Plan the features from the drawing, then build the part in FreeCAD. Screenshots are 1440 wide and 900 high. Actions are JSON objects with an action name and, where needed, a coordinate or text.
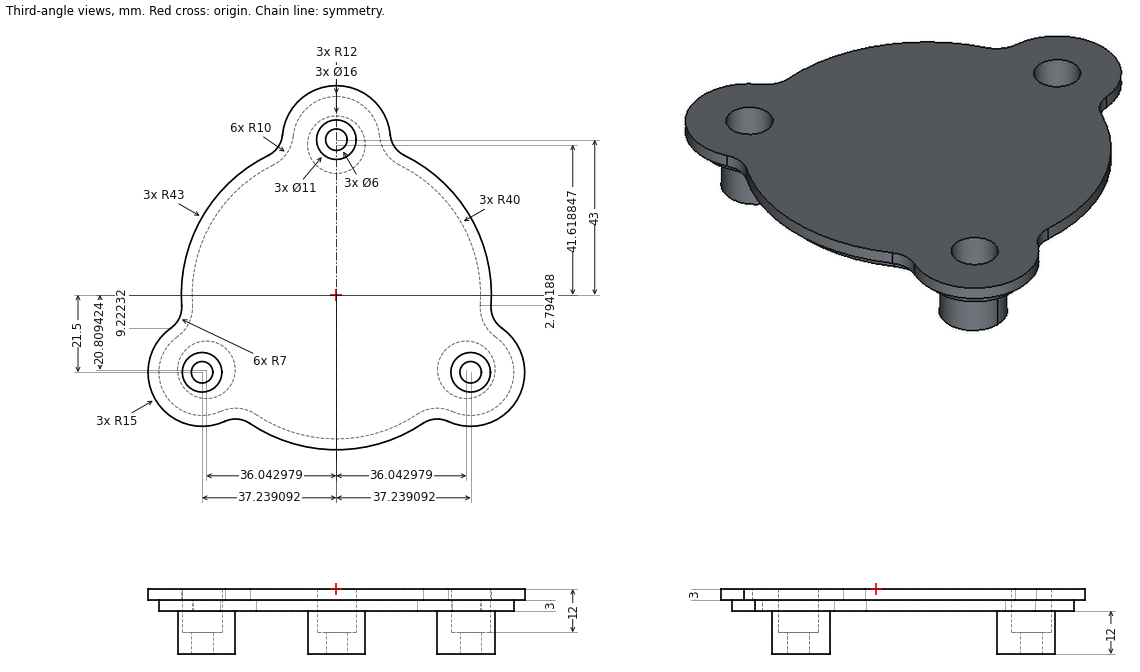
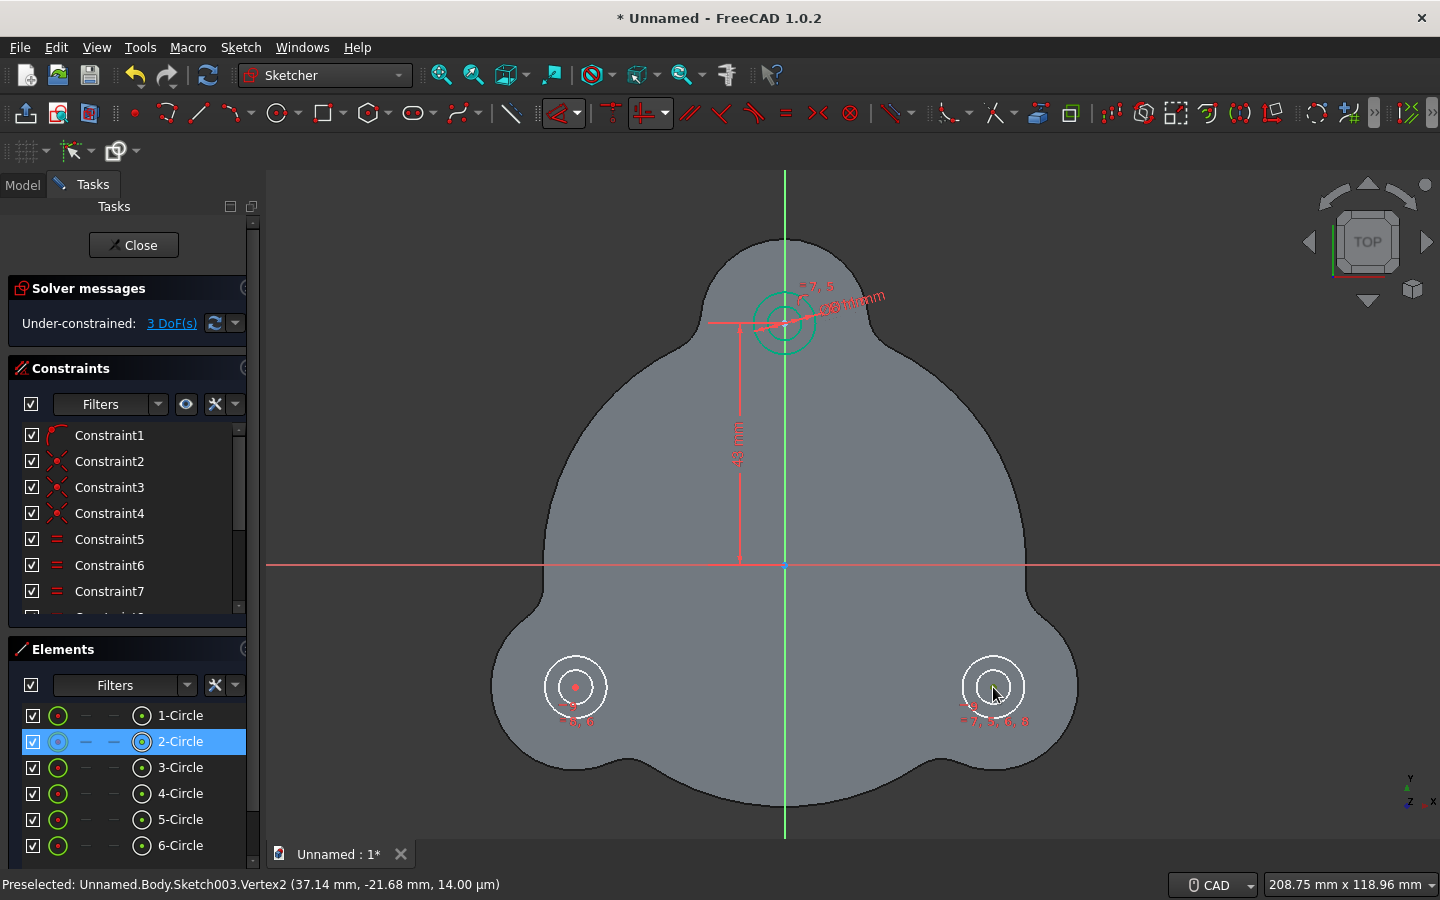
{"action": "left_click", "coordinate": [580, 114]}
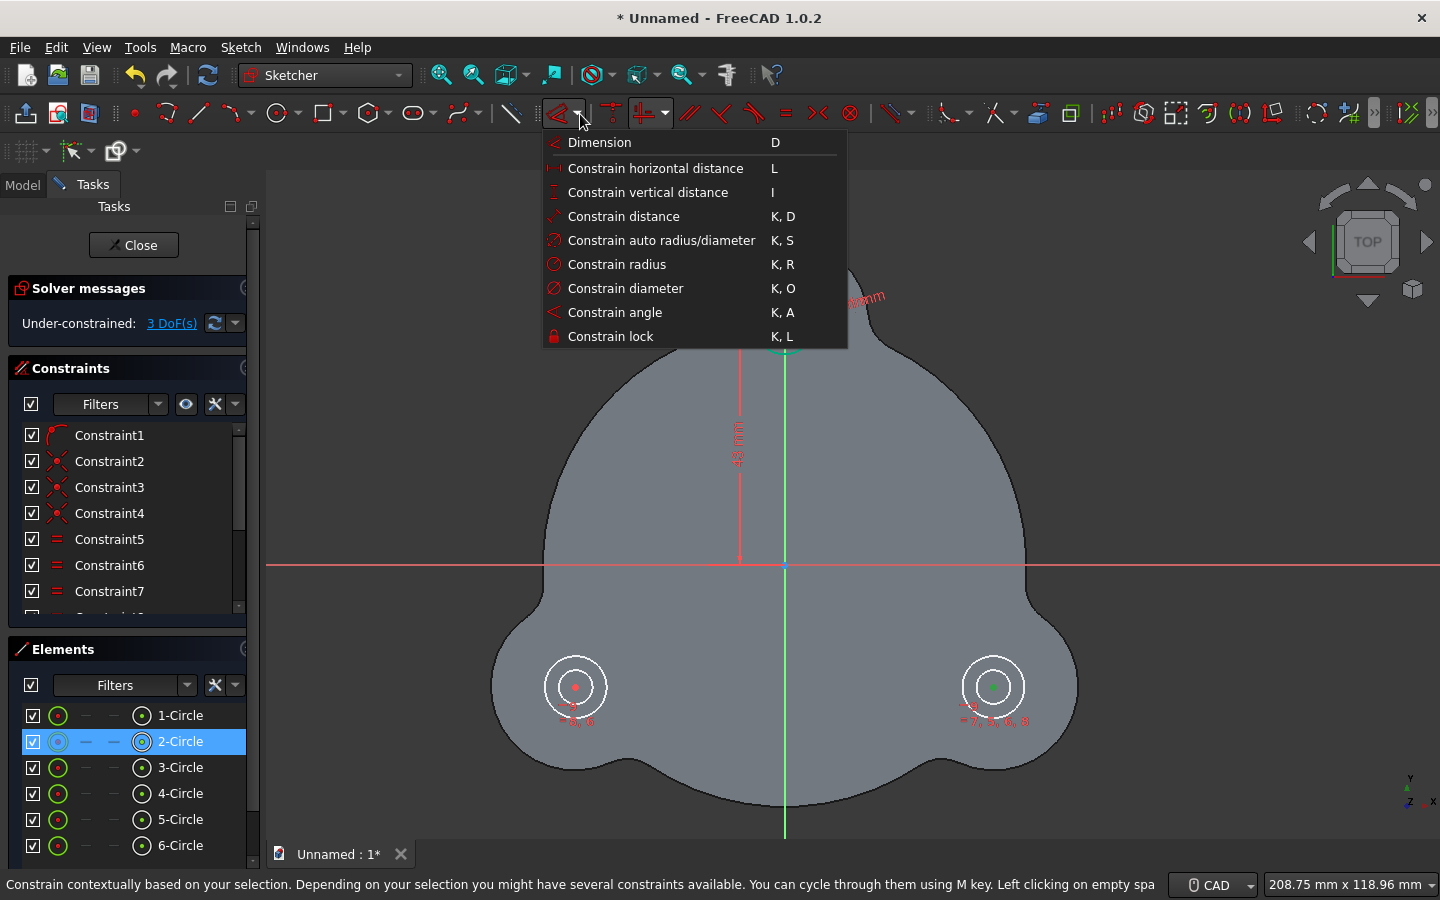
{"action": "left_click", "coordinate": [695, 192]}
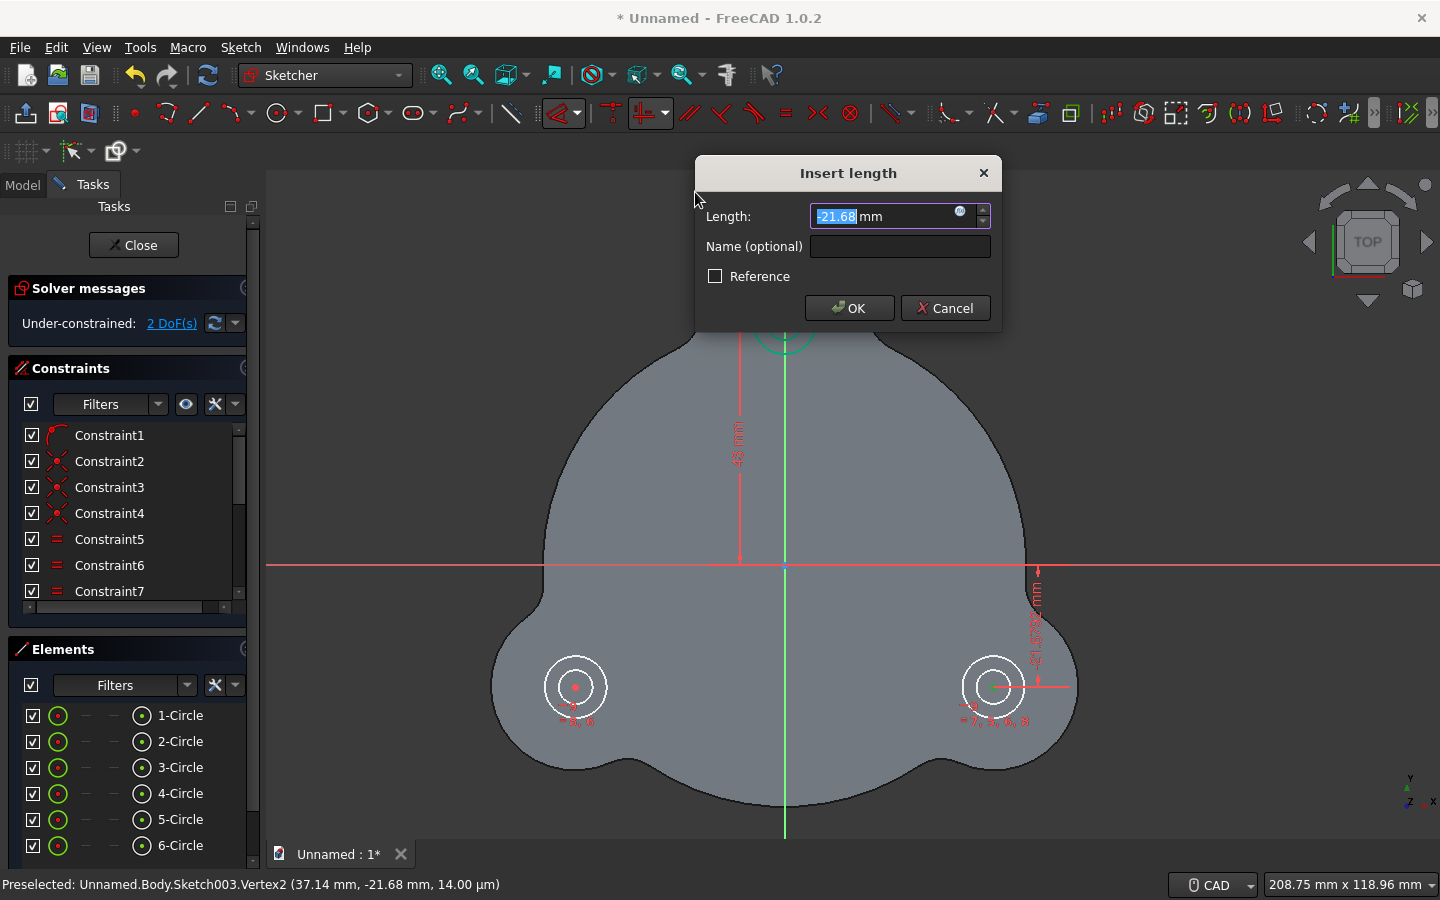
{"action": "type", "text": "-21.5"}
{"action": "key", "text": "Return"}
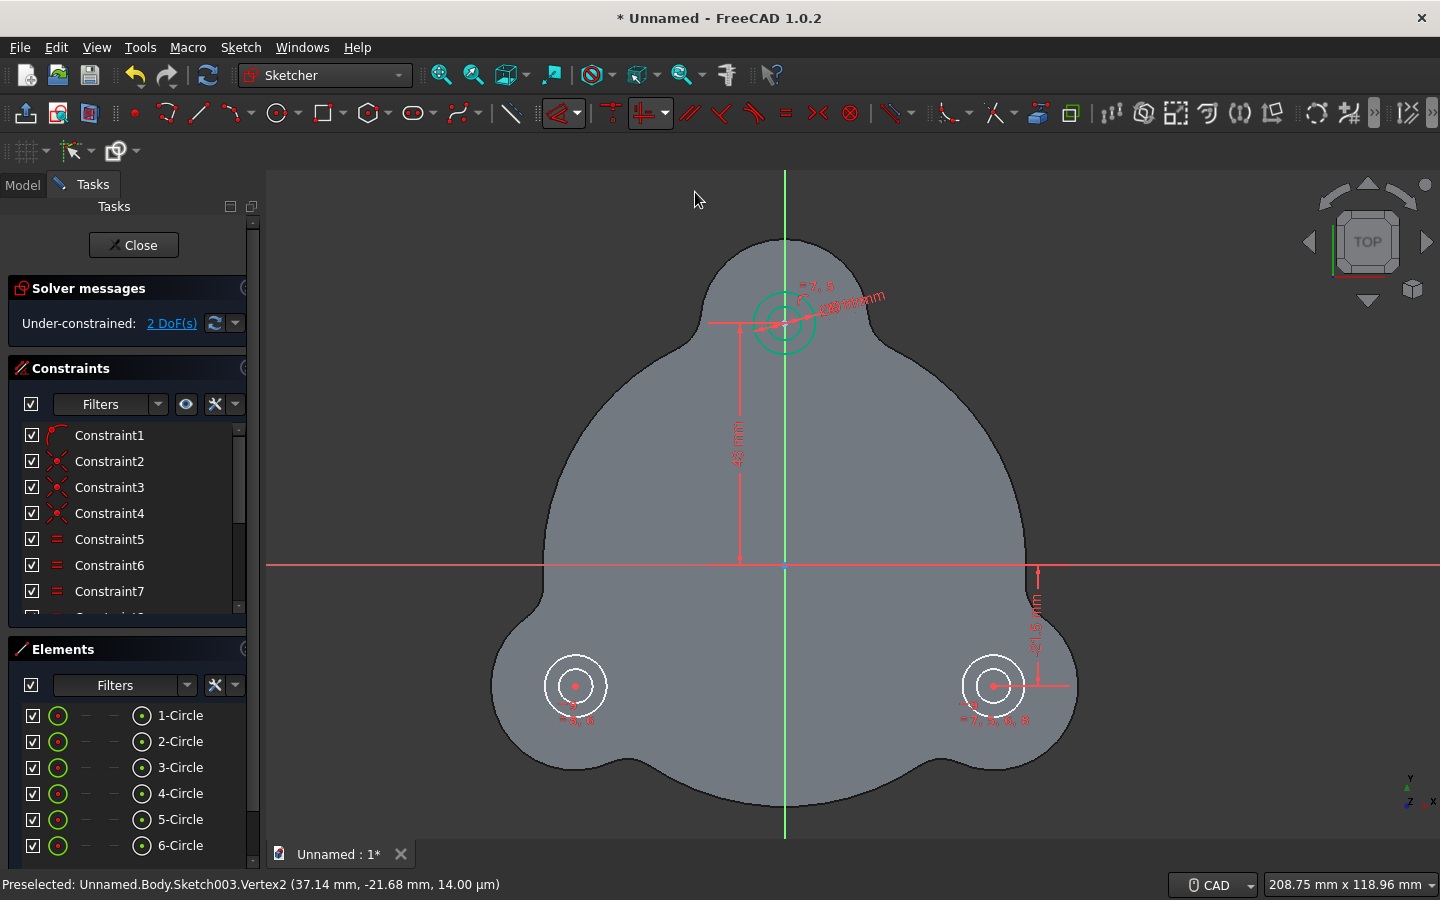
{"action": "left_click", "coordinate": [993, 686]}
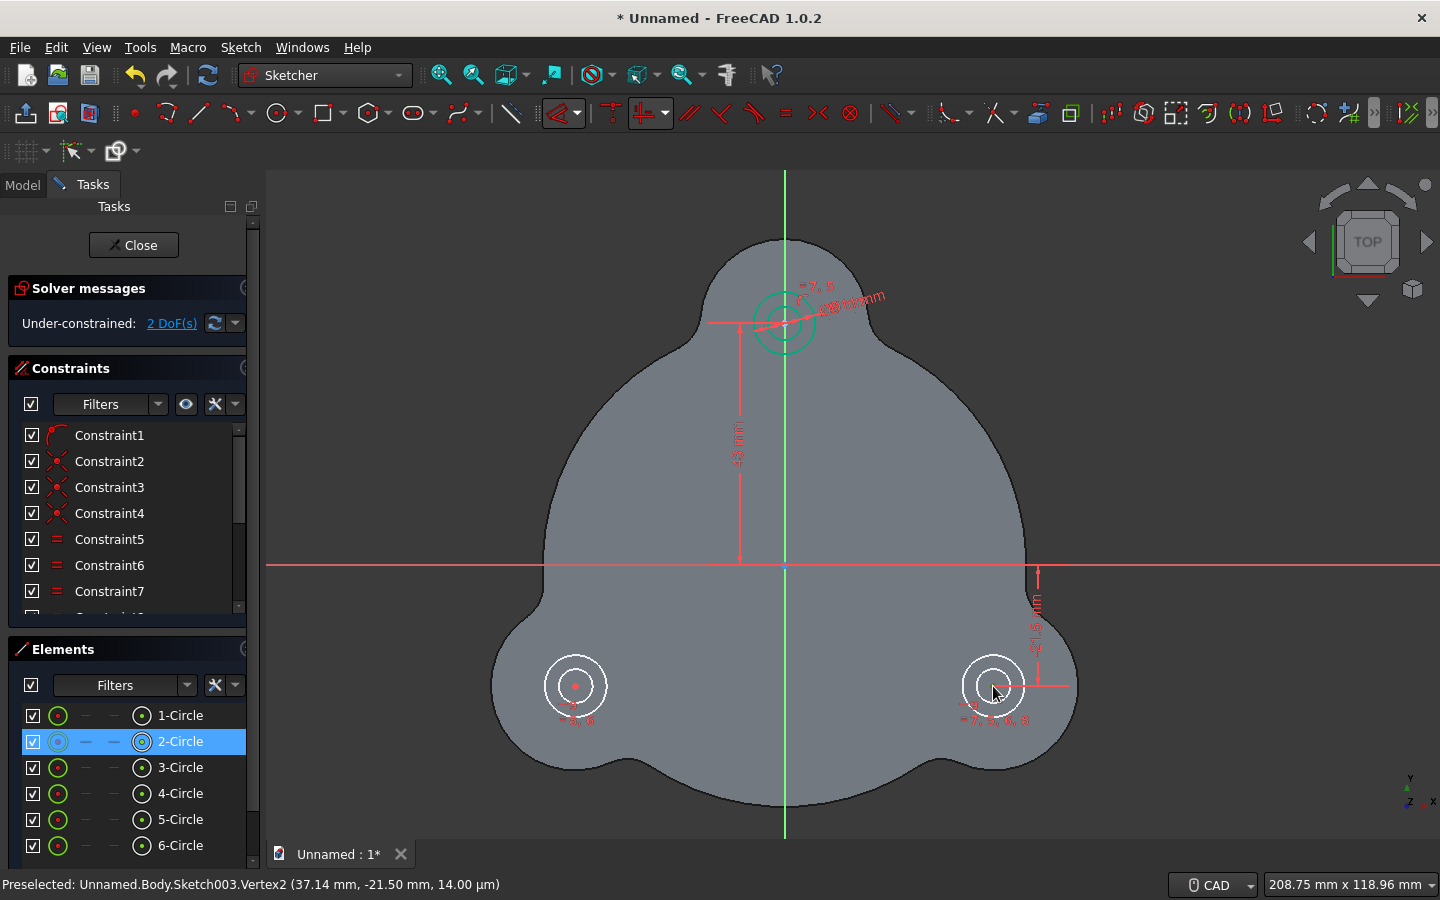
{"action": "left_click", "coordinate": [580, 114]}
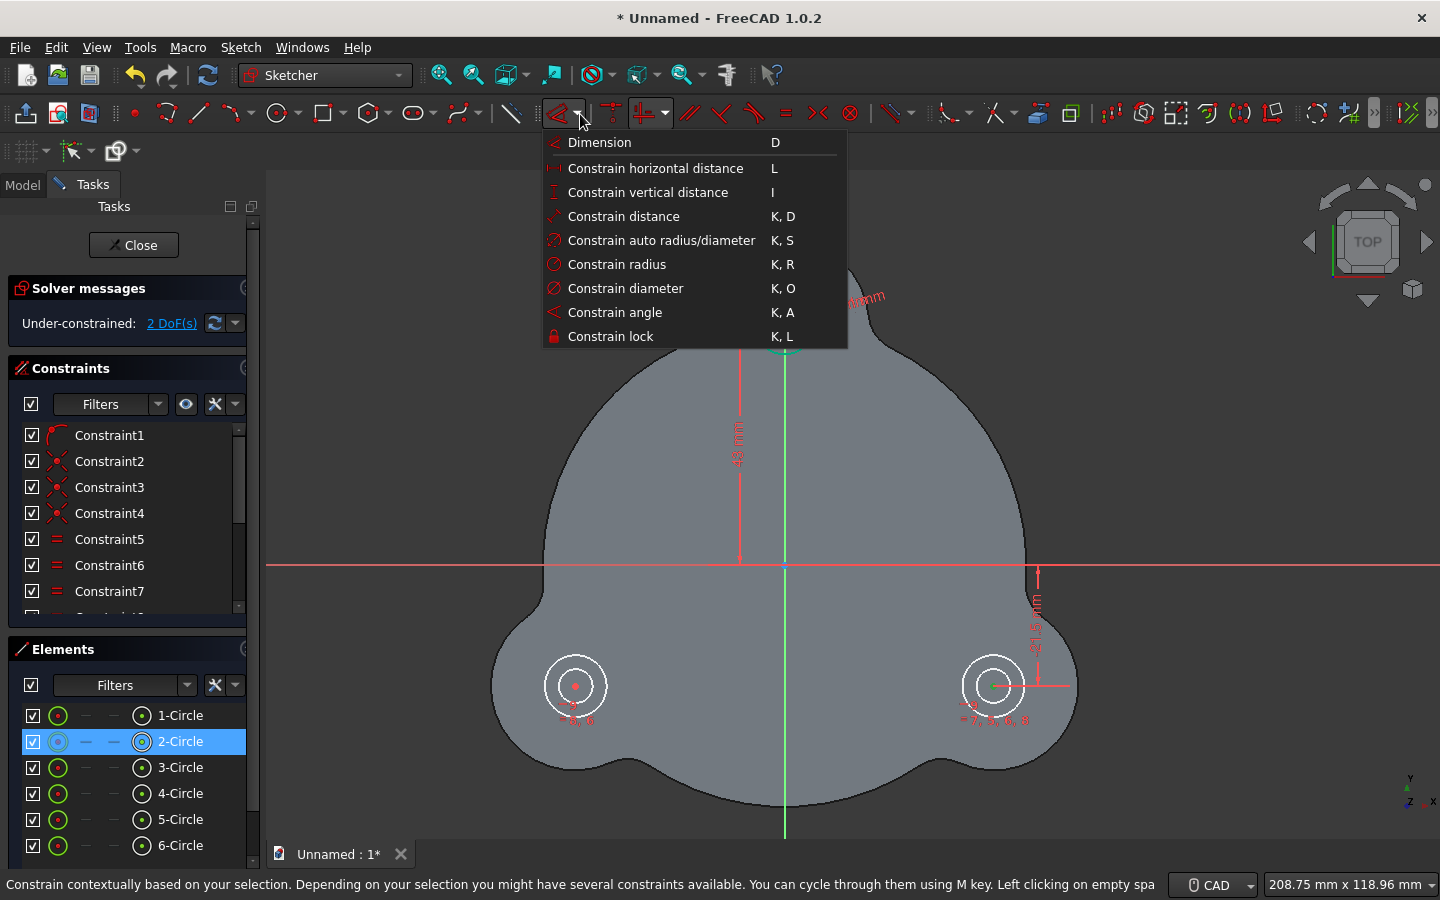
{"action": "left_click", "coordinate": [695, 168]}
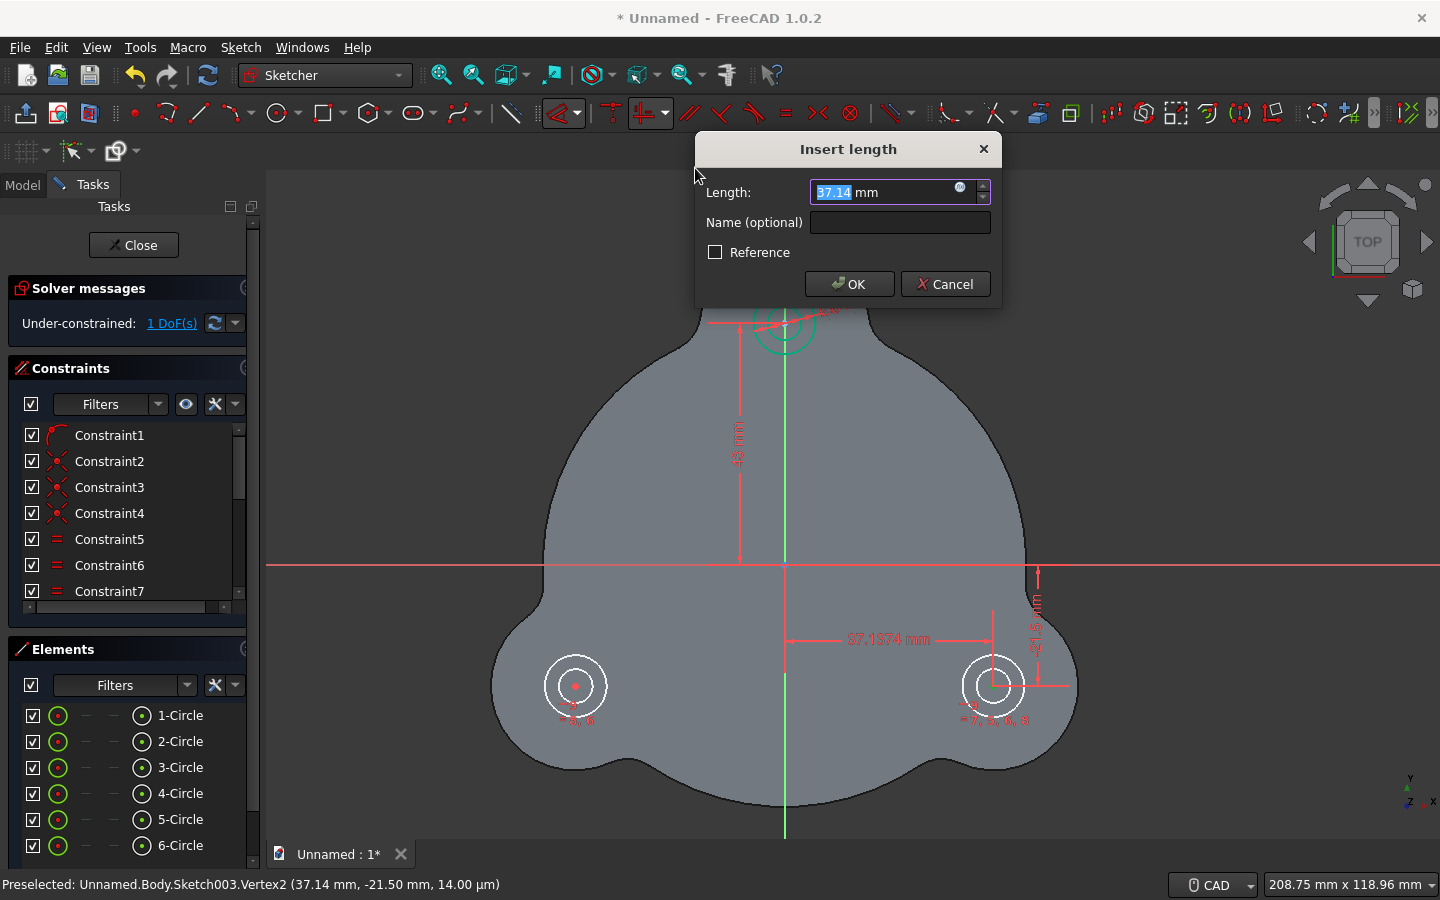
{"action": "type", "text": "37.239092"}
{"action": "key", "text": "Return"}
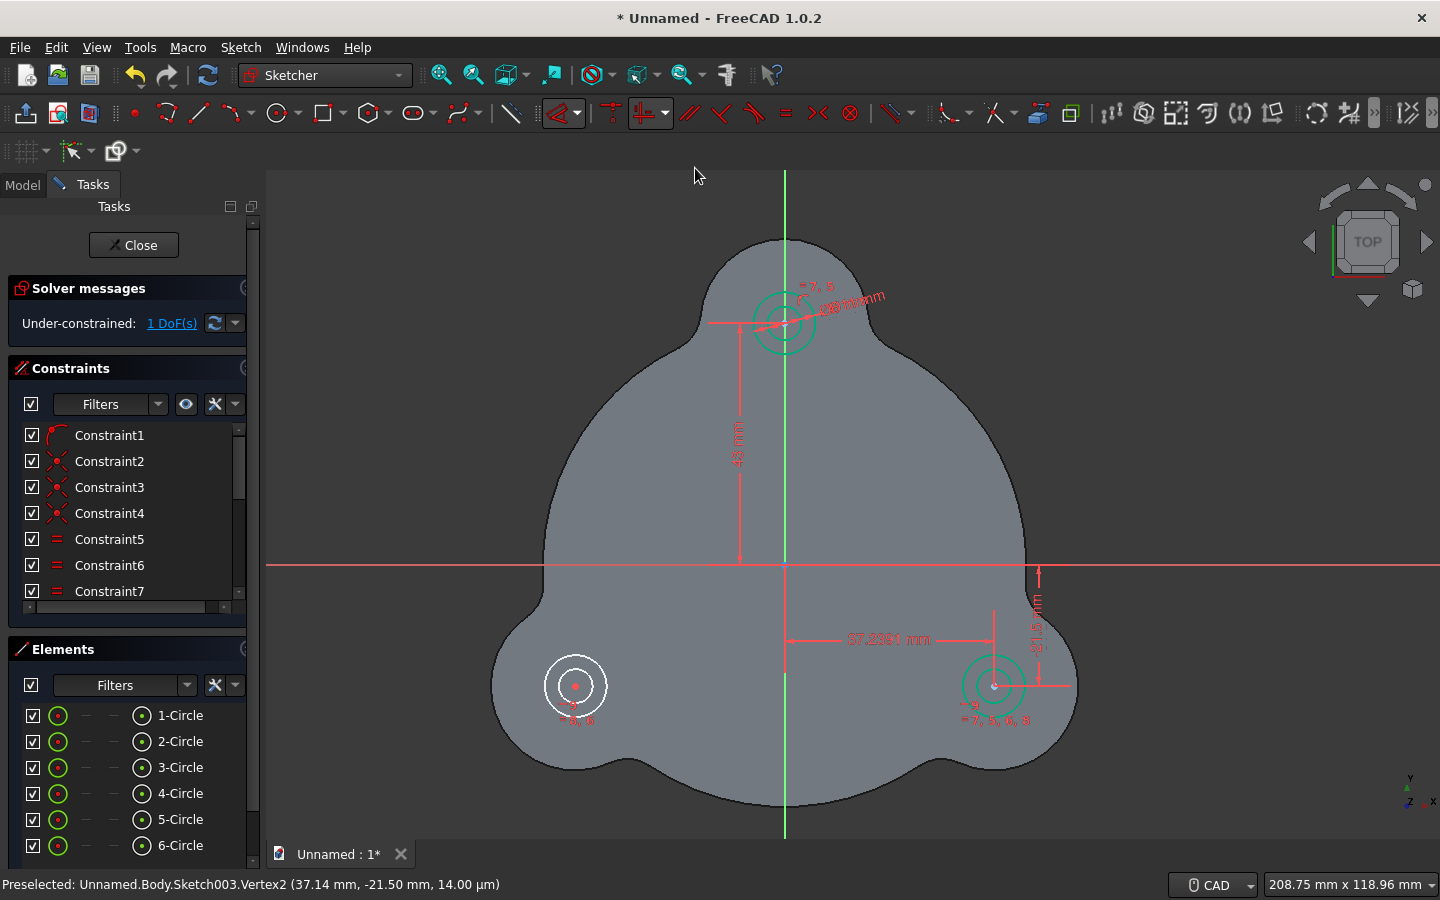
{"action": "left_click", "coordinate": [576, 686]}